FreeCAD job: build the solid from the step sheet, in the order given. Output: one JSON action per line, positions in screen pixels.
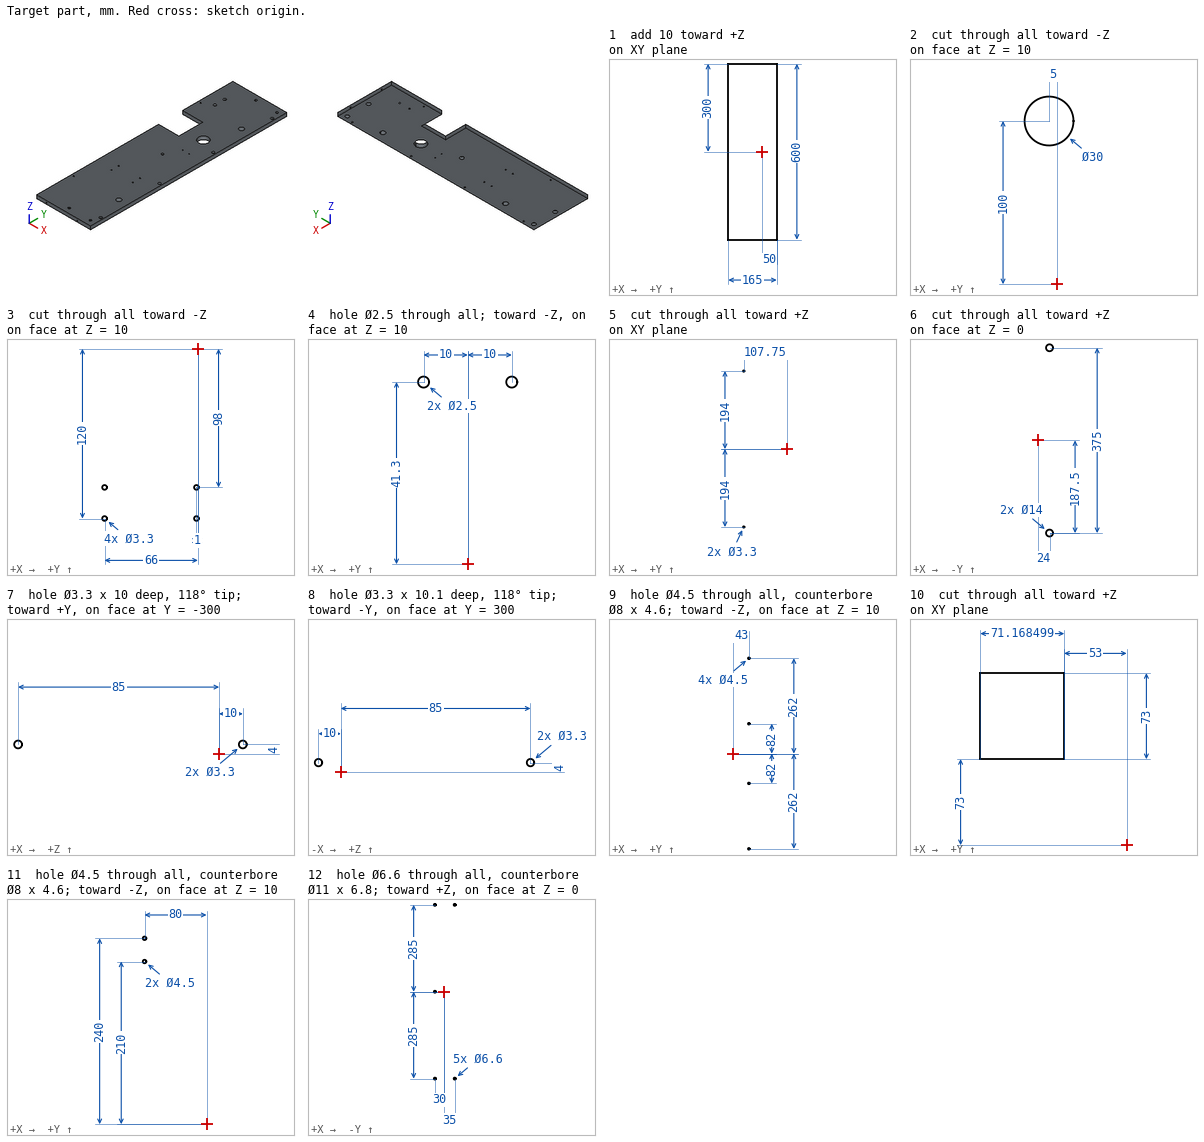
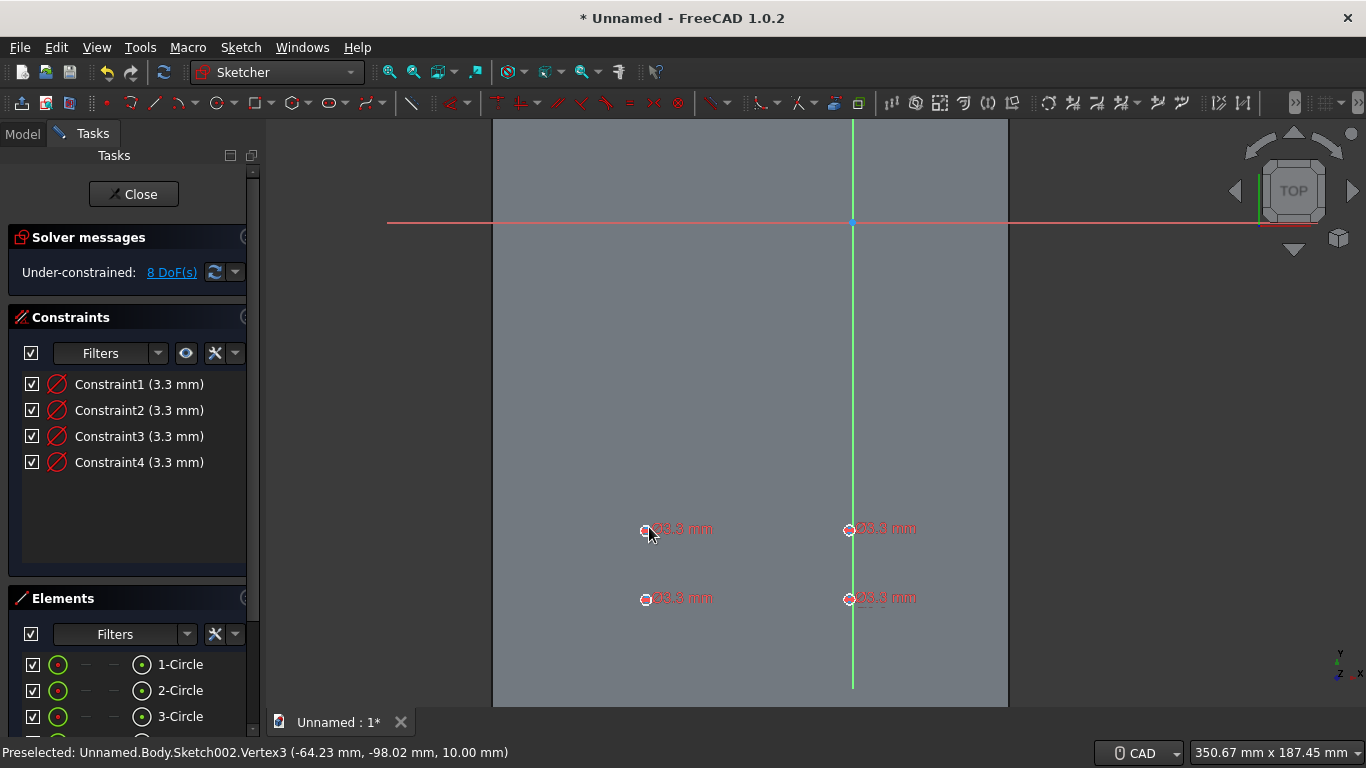
{"action": "left_click", "coordinate": [849, 530]}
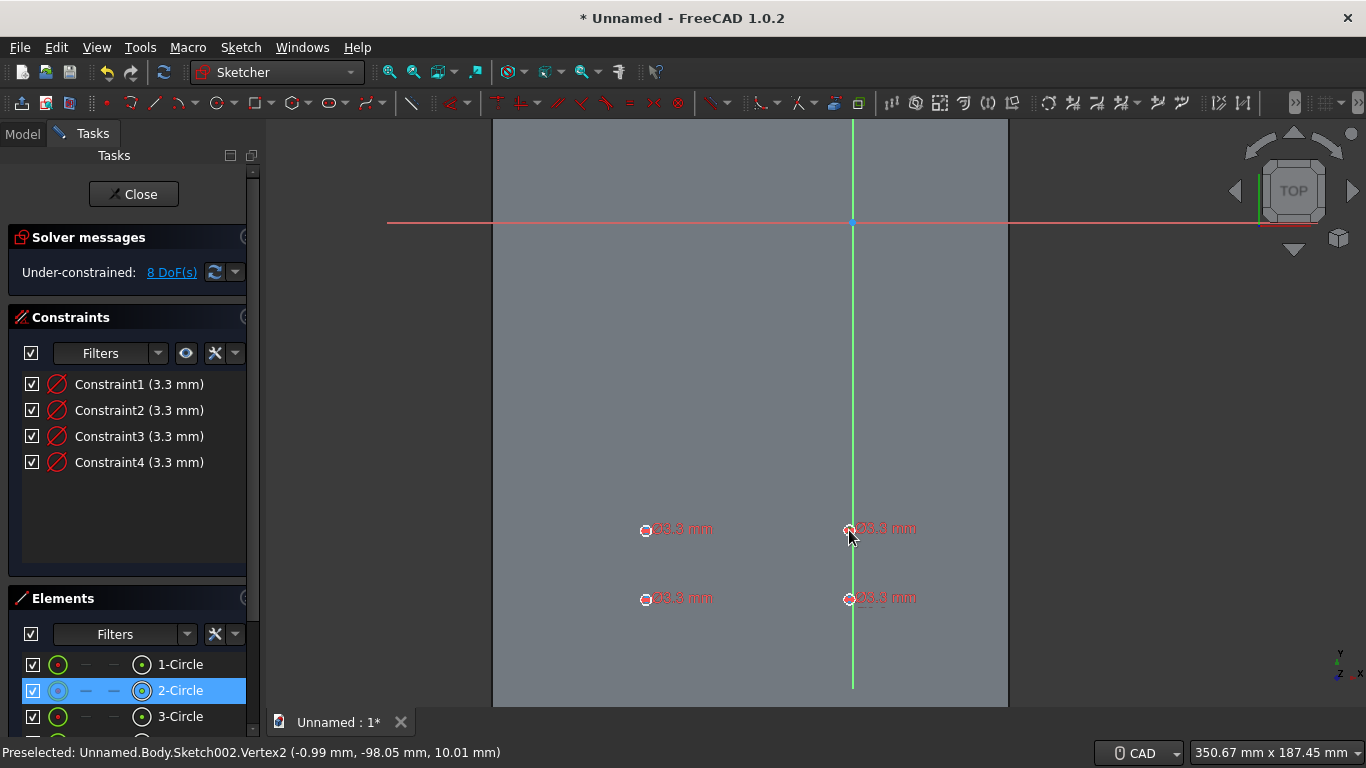
{"action": "left_click", "coordinate": [849, 600]}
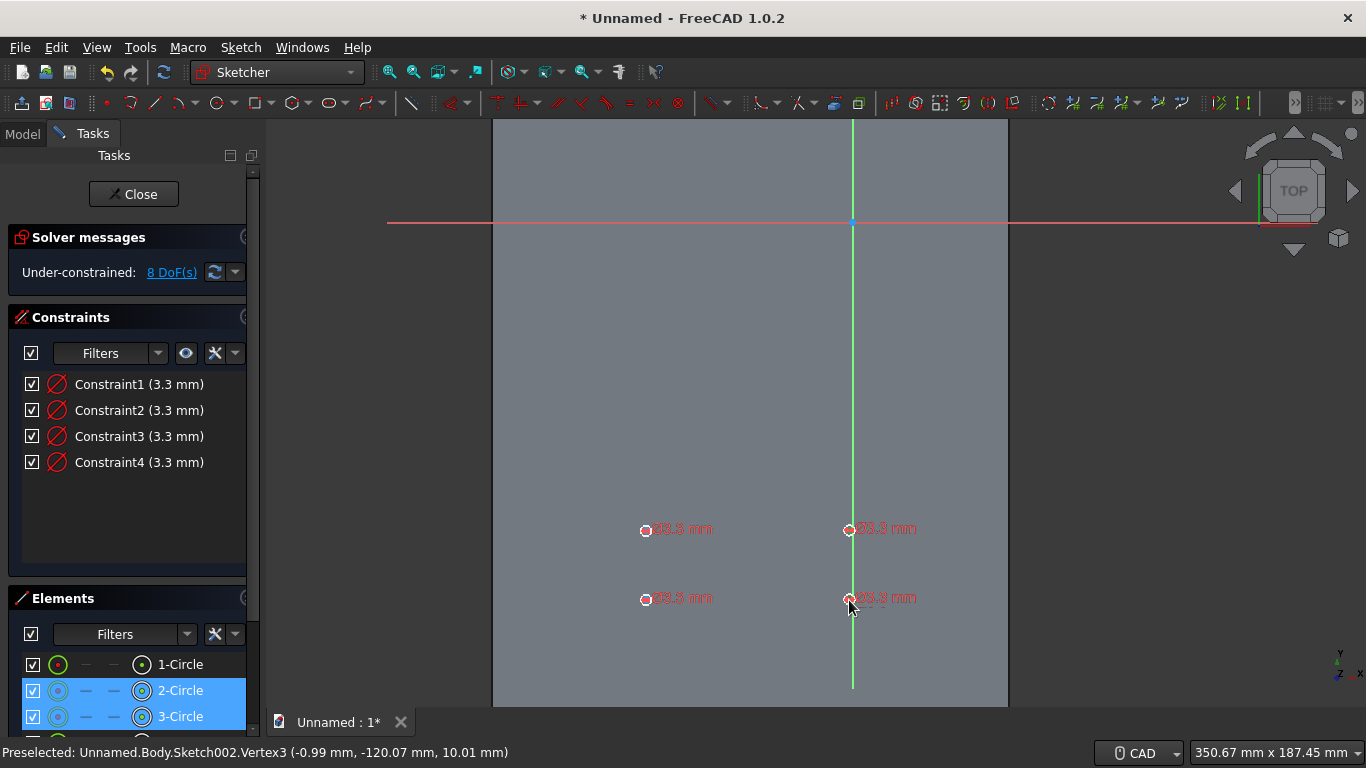
{"action": "left_click", "coordinate": [540, 104]}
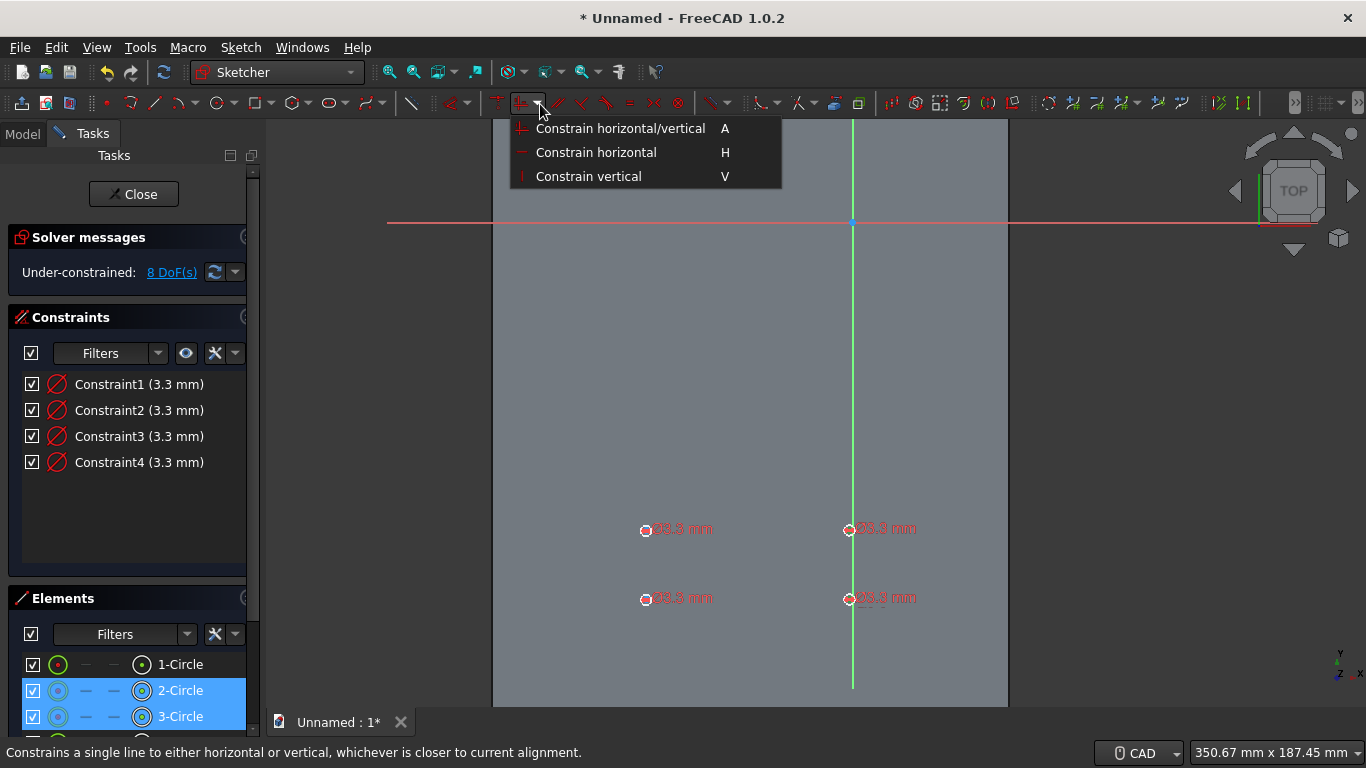
{"action": "left_click", "coordinate": [646, 176]}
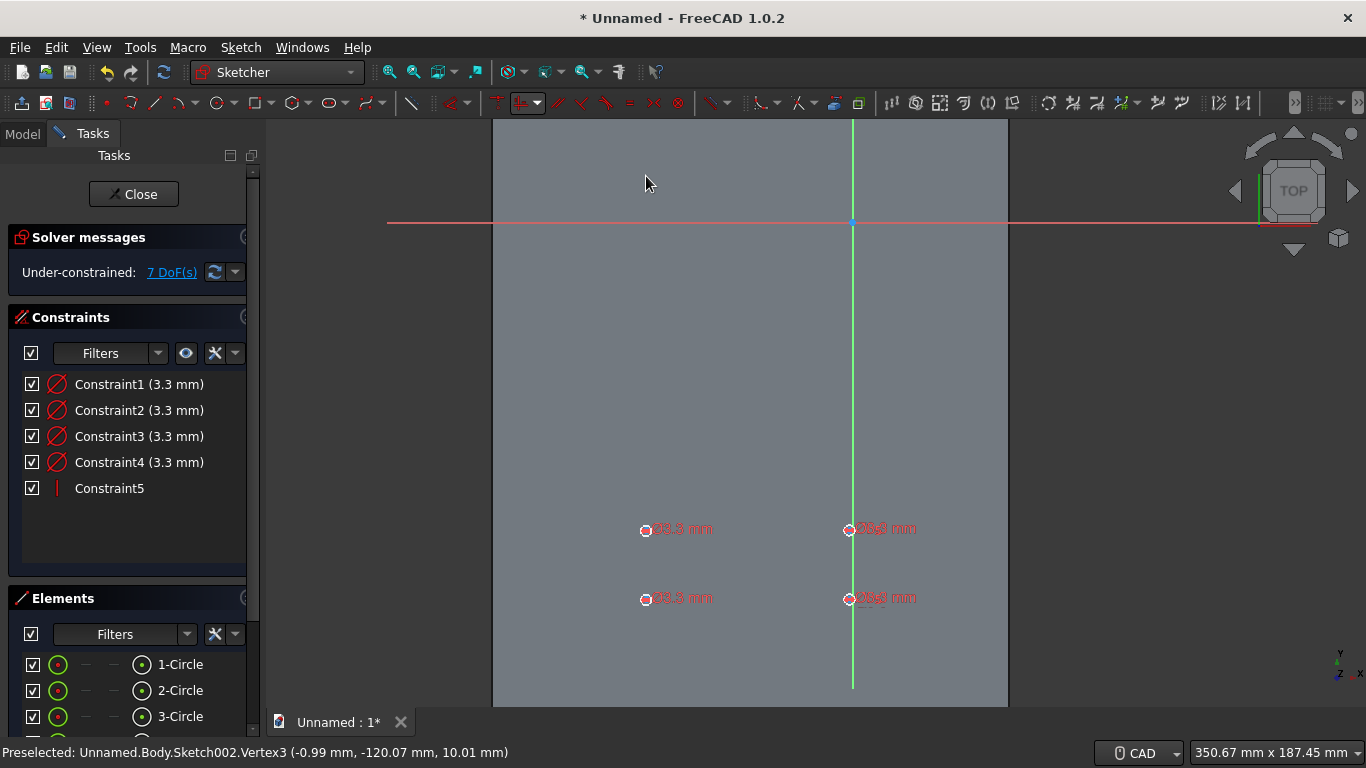
{"action": "left_click", "coordinate": [646, 600]}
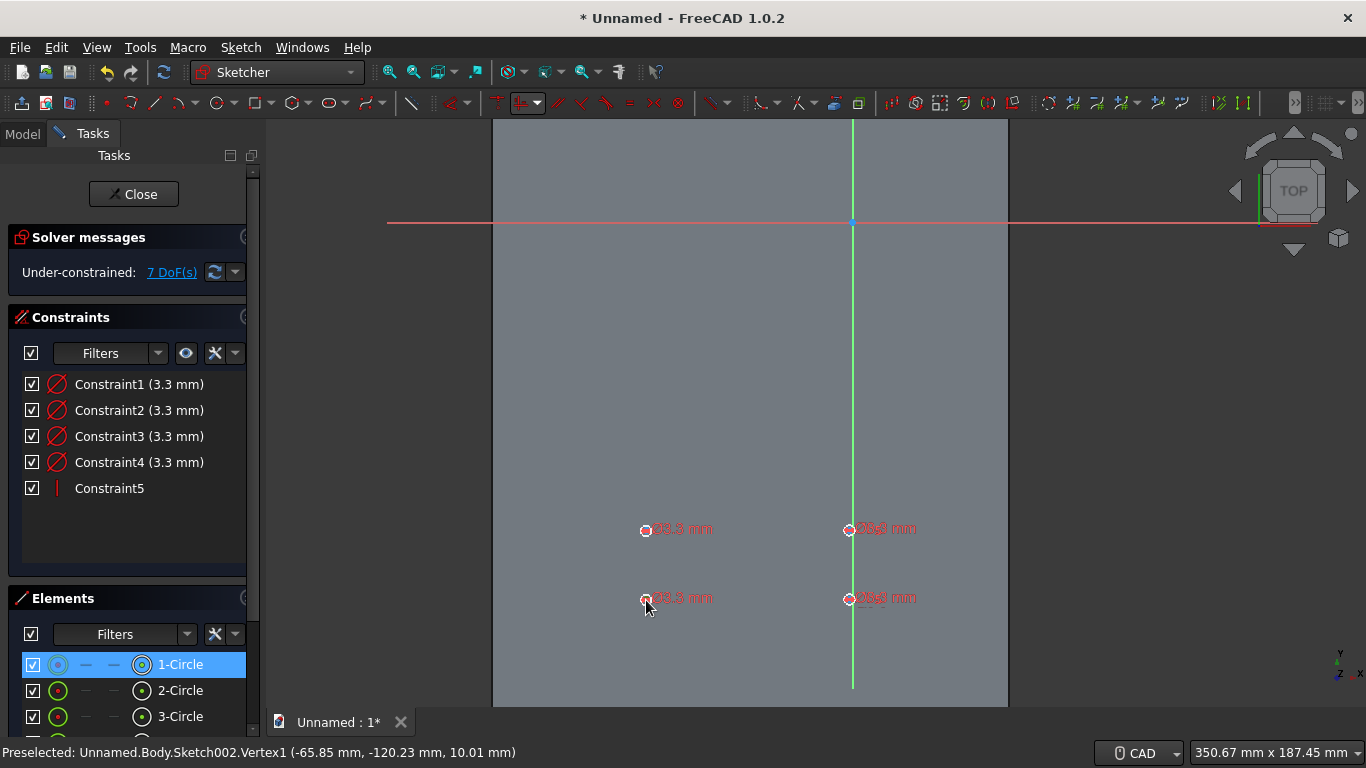
{"action": "left_click", "coordinate": [849, 600]}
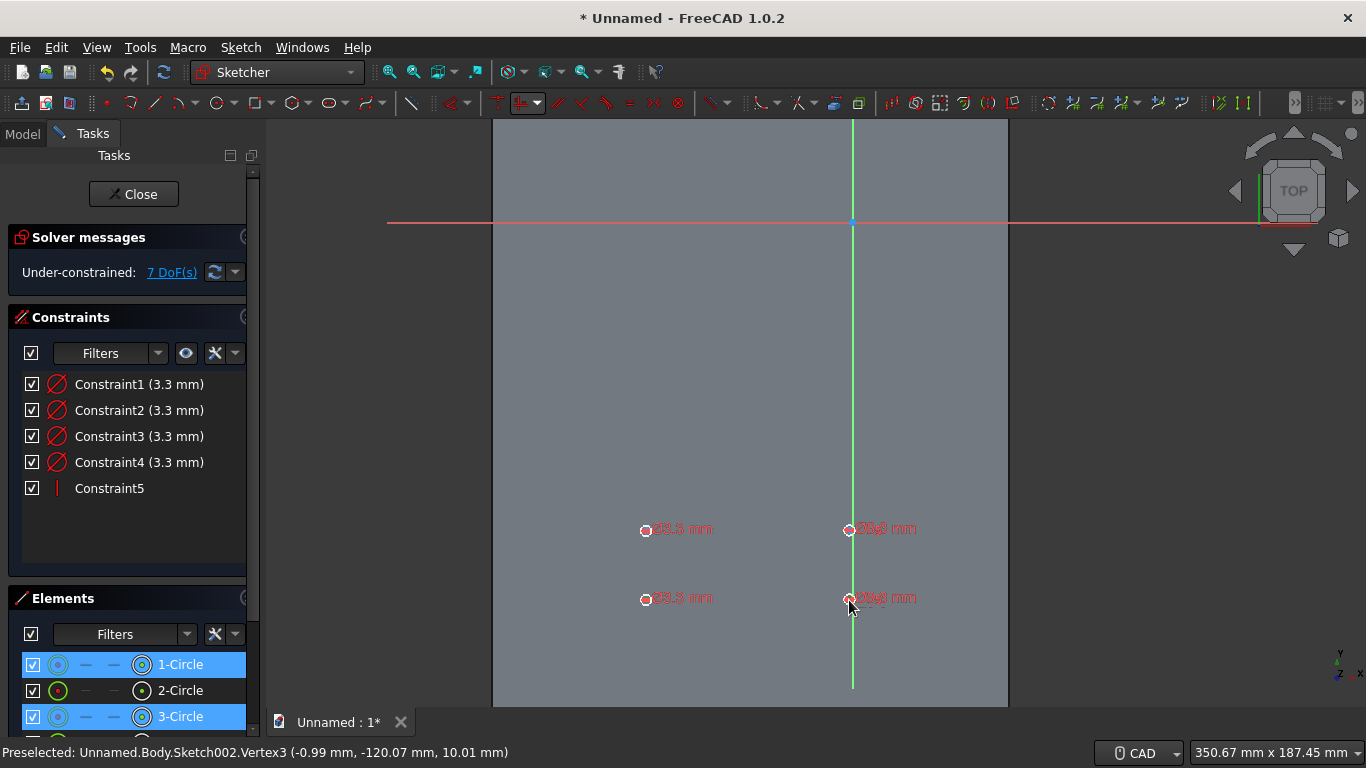
{"action": "key", "text": "h"}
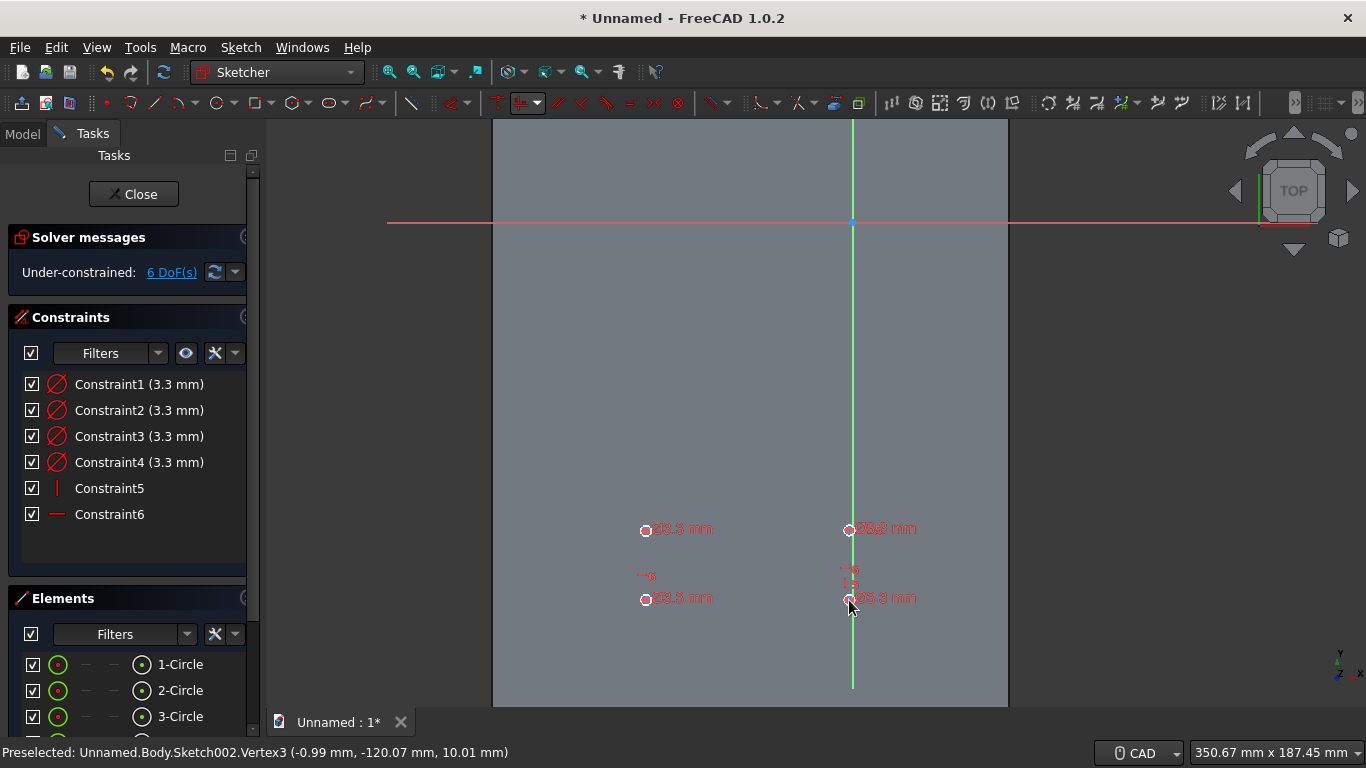
{"action": "left_click", "coordinate": [646, 600]}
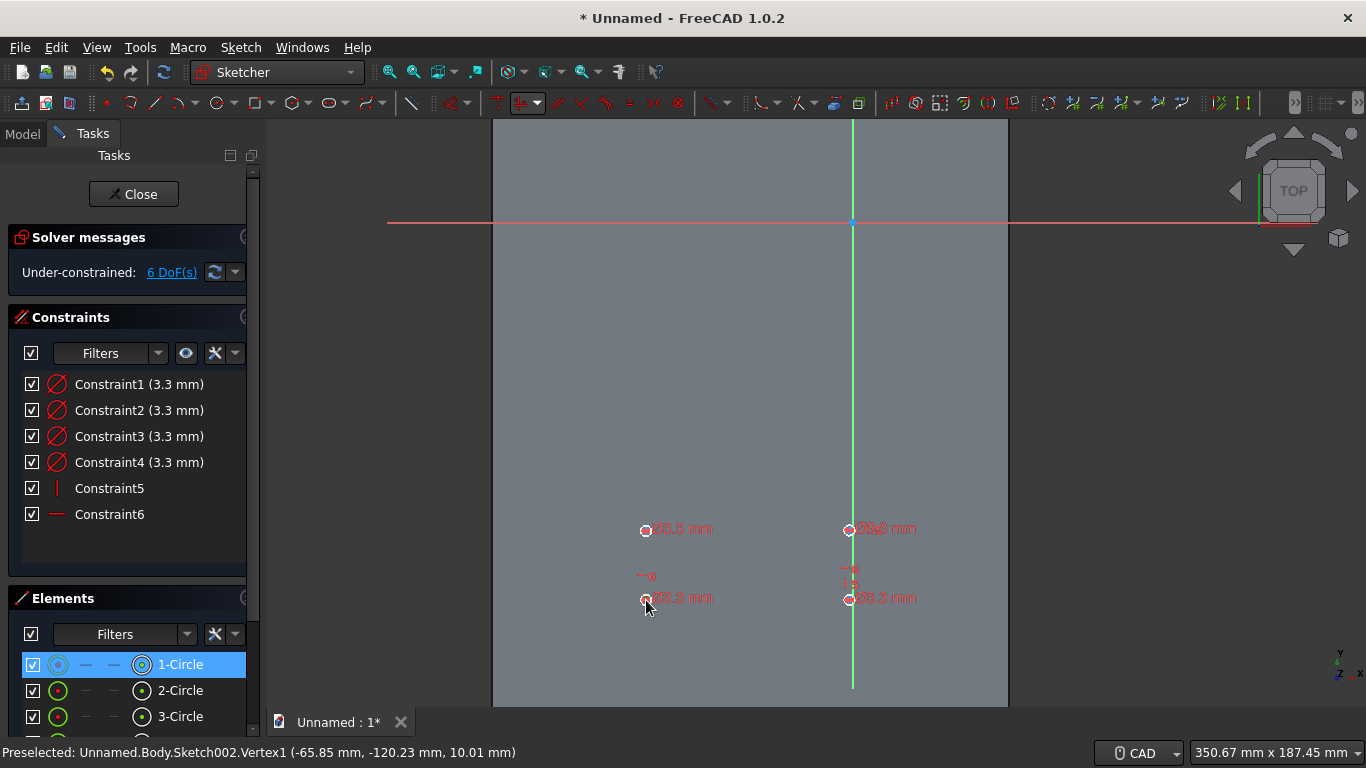
{"action": "left_click", "coordinate": [646, 531]}